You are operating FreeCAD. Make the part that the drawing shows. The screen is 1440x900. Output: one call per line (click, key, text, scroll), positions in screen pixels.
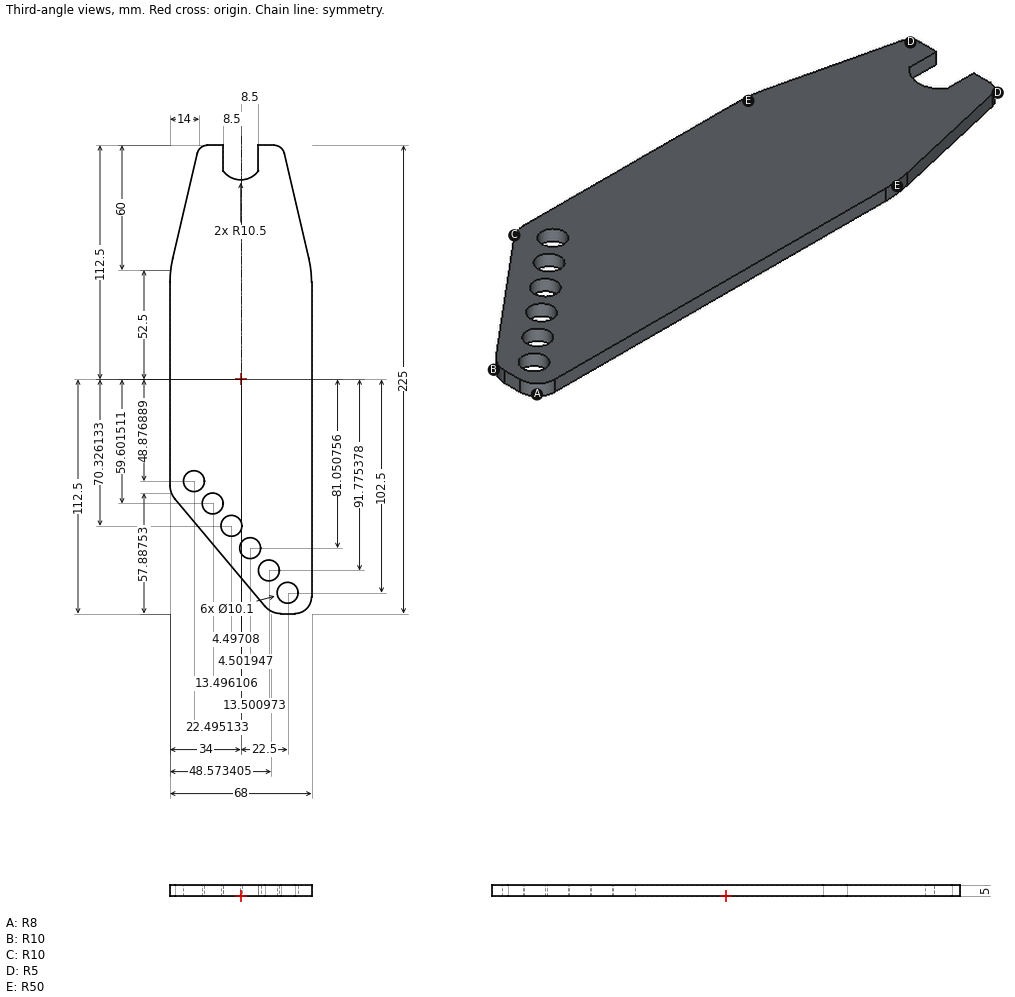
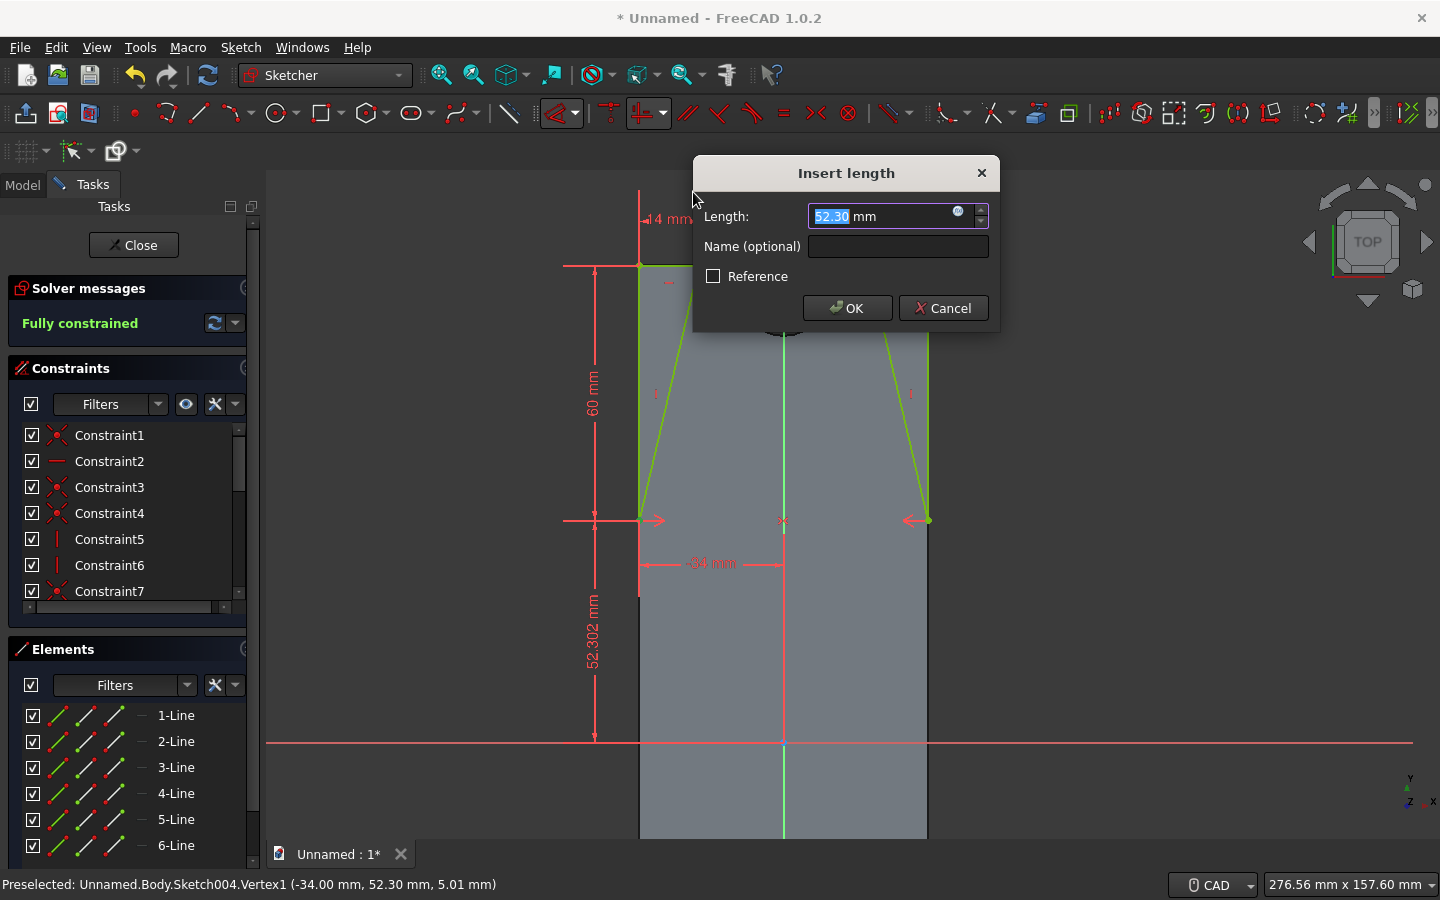
text(52.5)
key(Return)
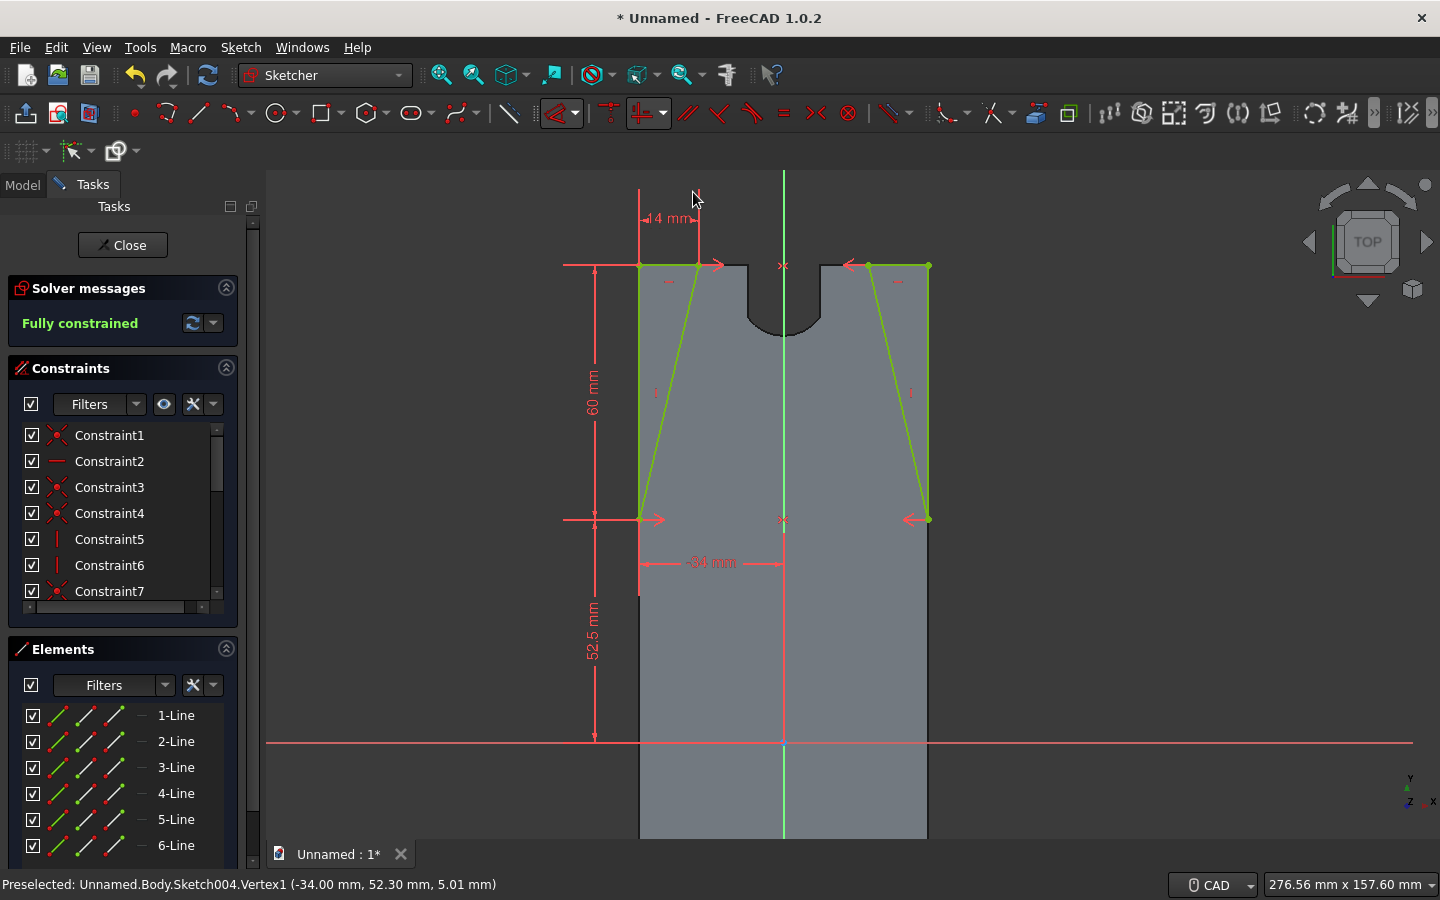
click(123, 245)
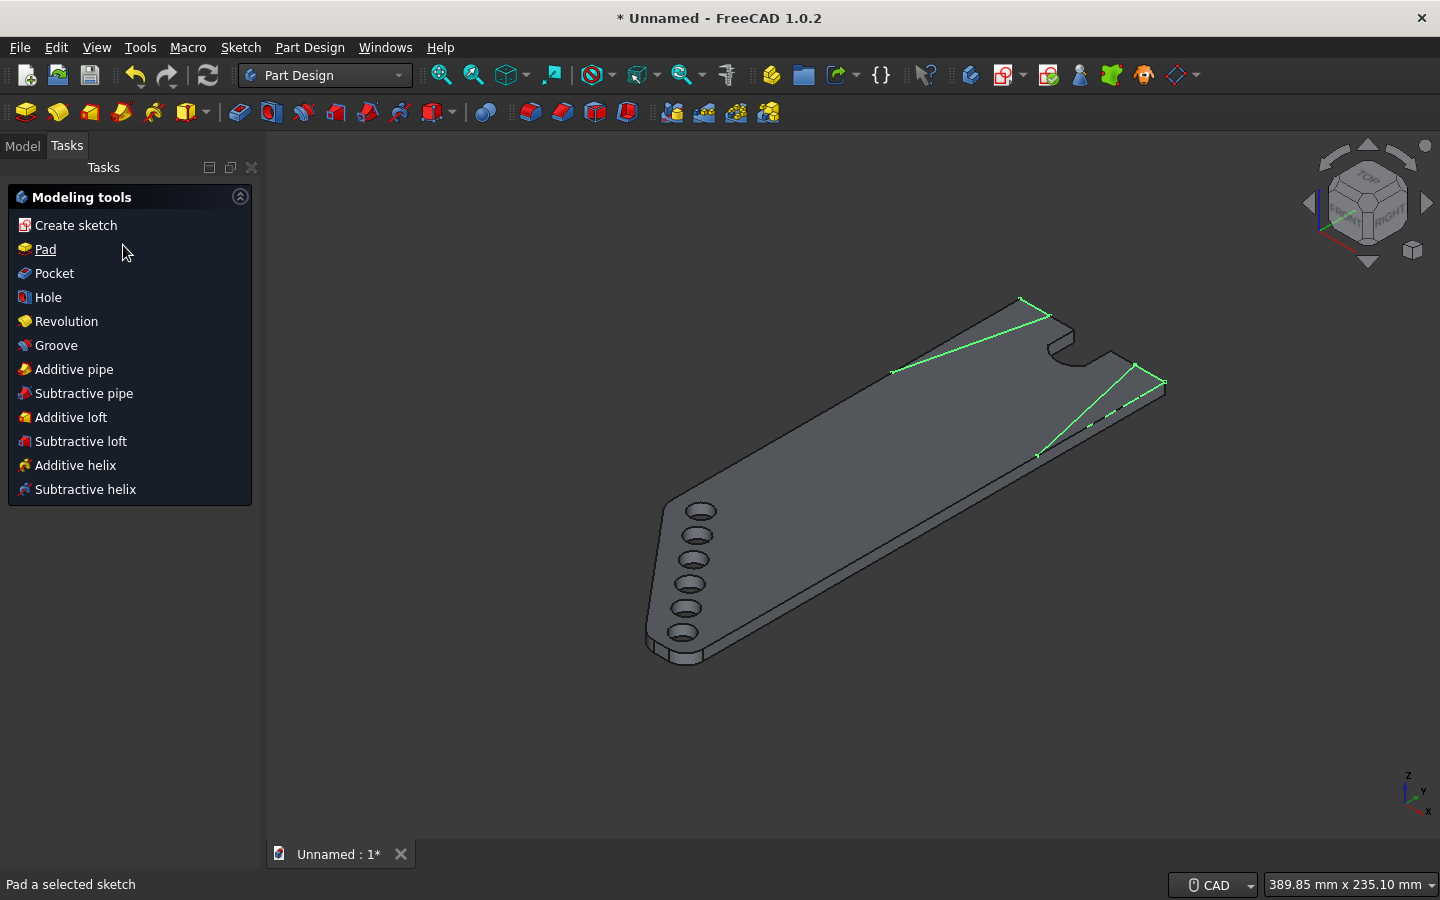
click(240, 112)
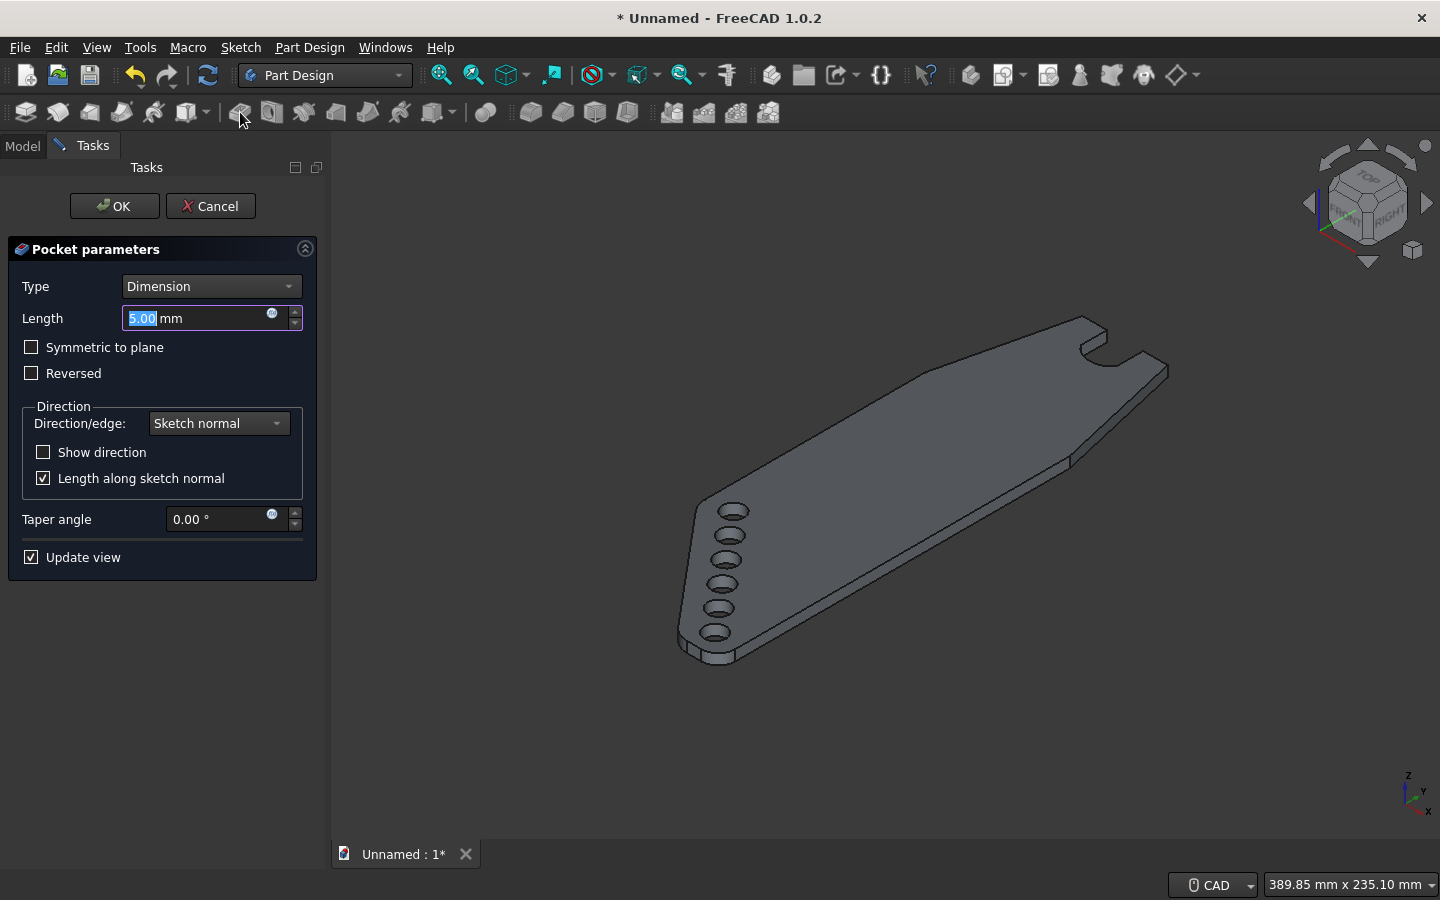
click(212, 286)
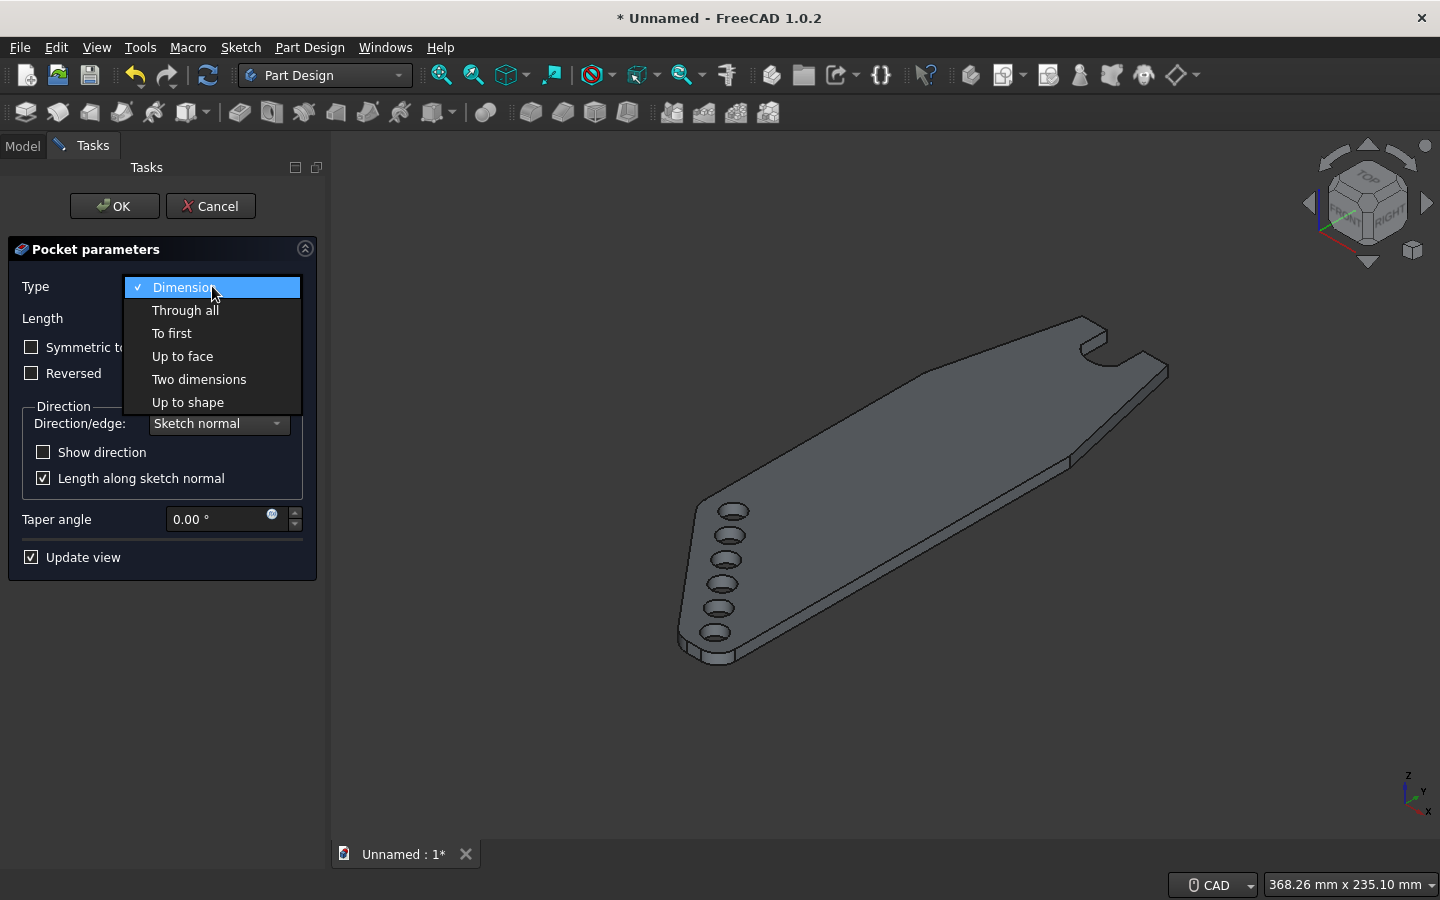
click(212, 310)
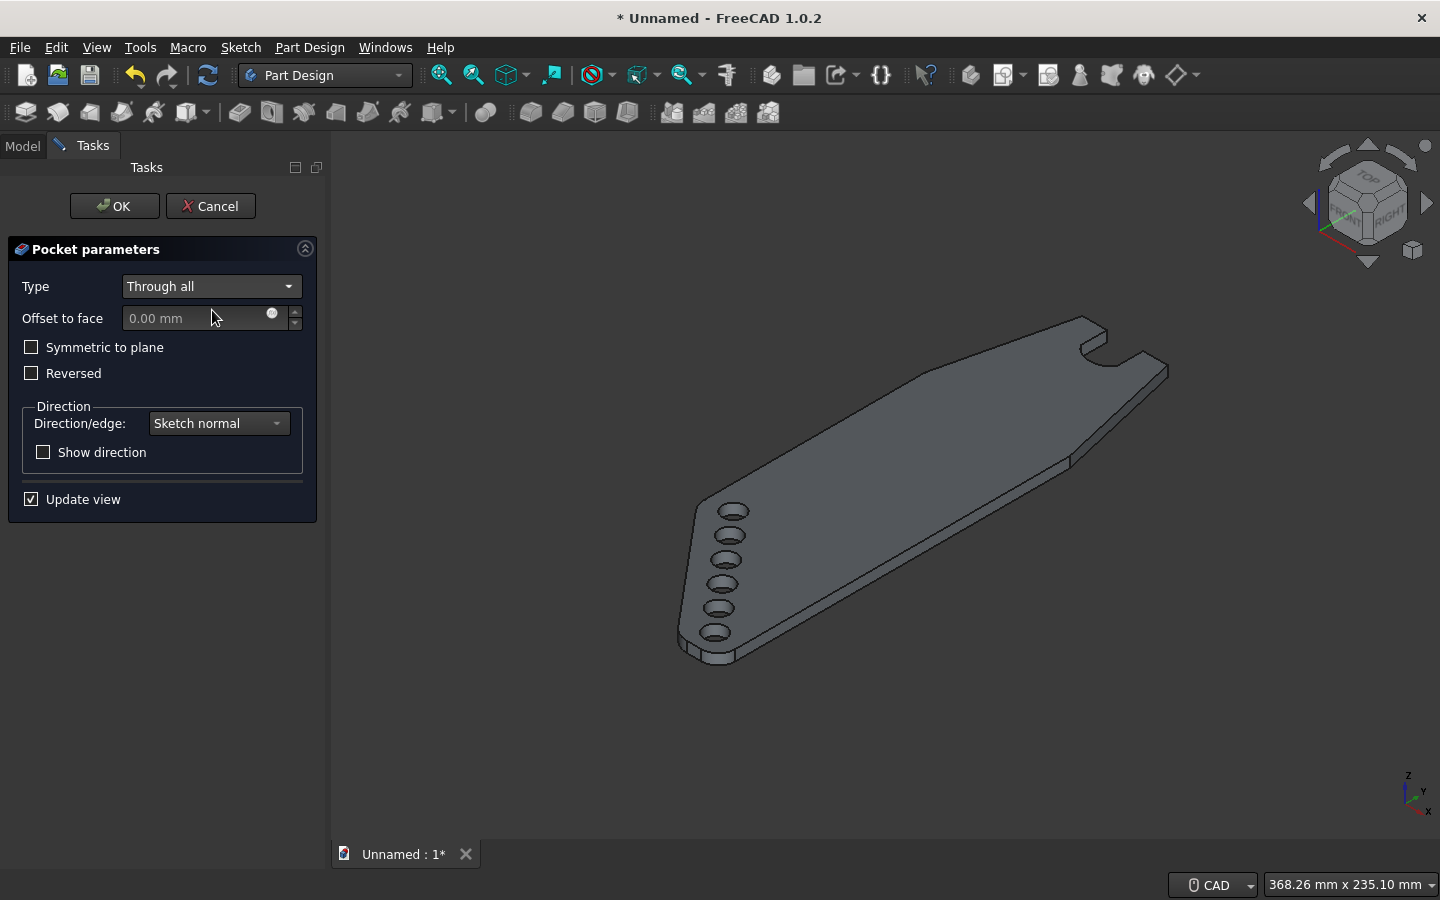
click(115, 206)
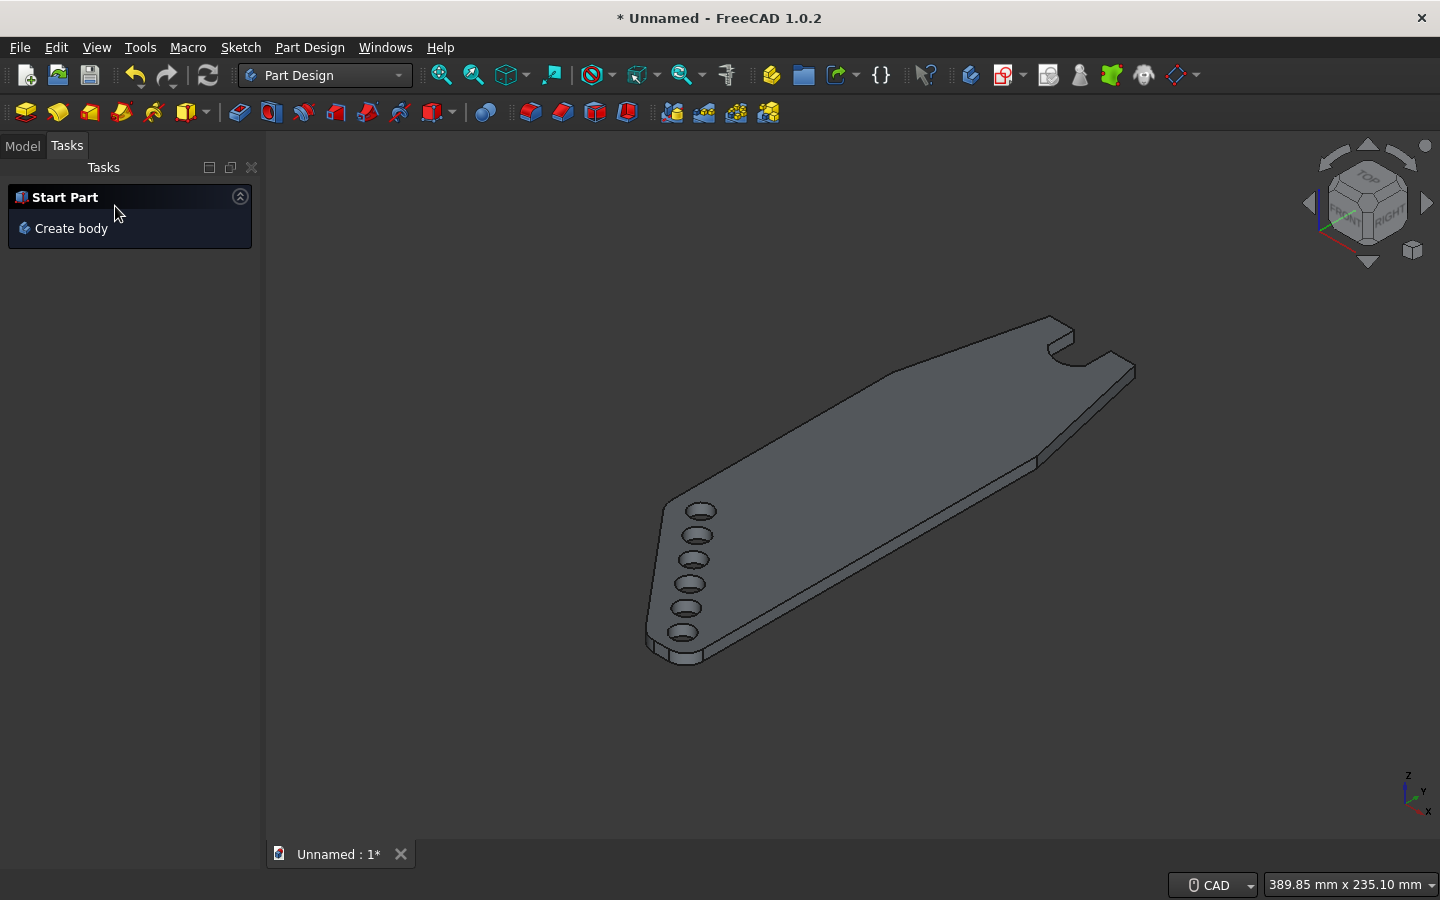
scroll(1050, 321, up, 5)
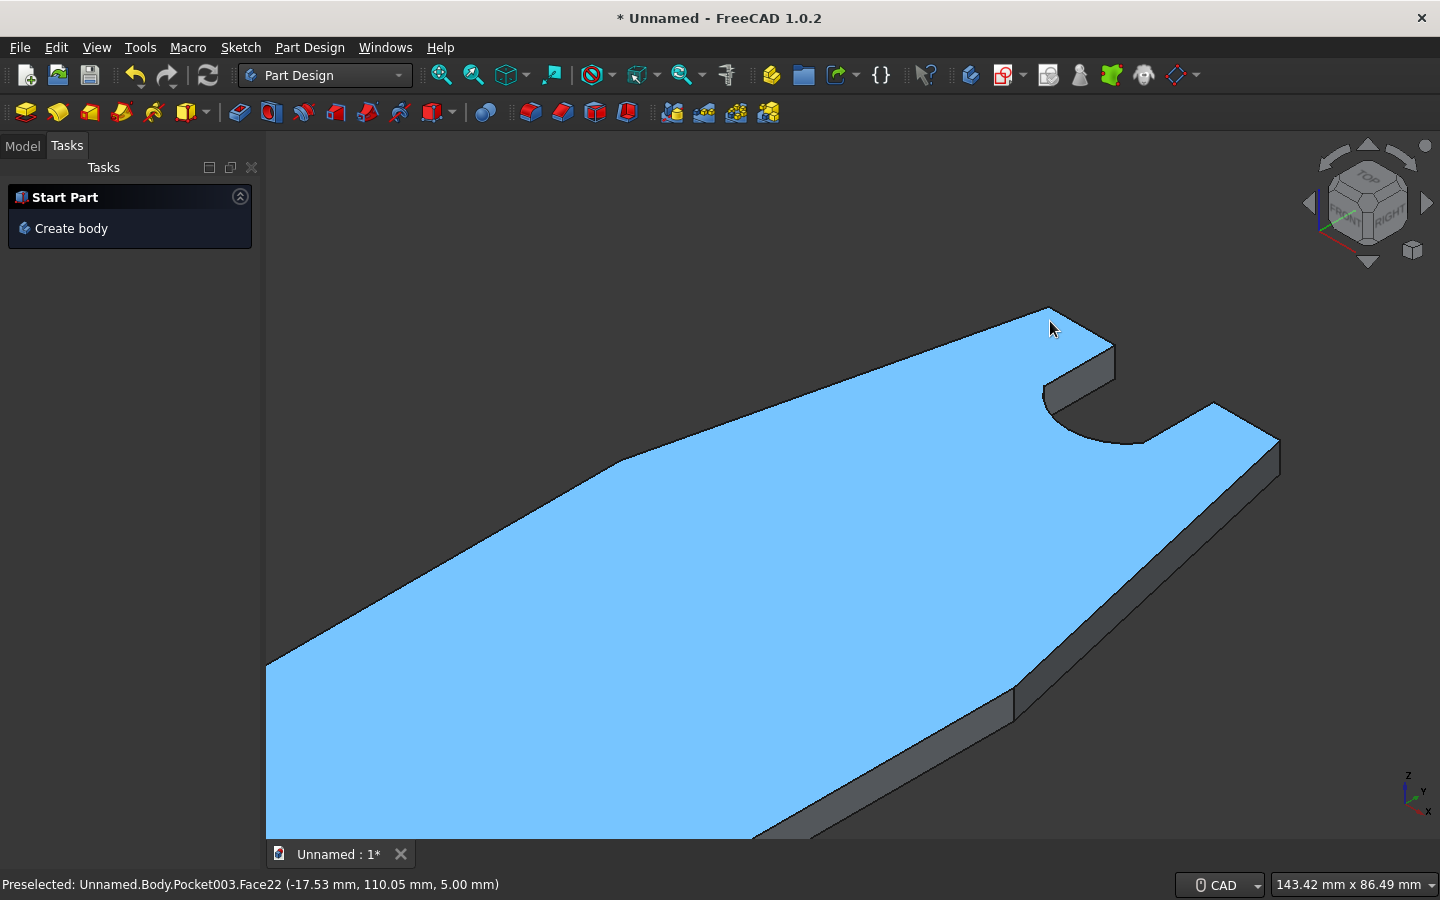
key(v)
key(f)